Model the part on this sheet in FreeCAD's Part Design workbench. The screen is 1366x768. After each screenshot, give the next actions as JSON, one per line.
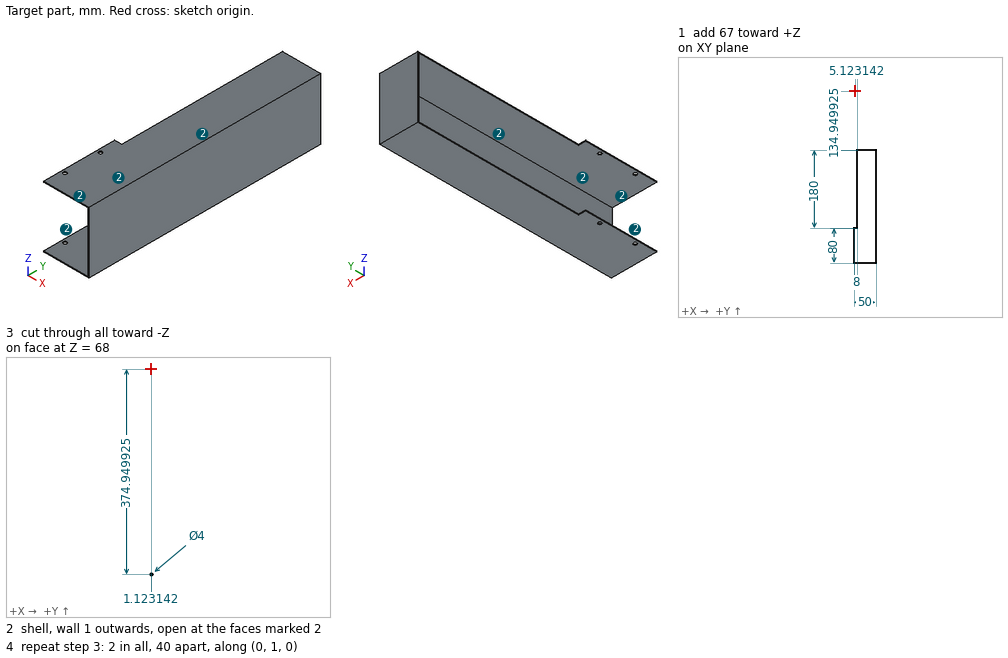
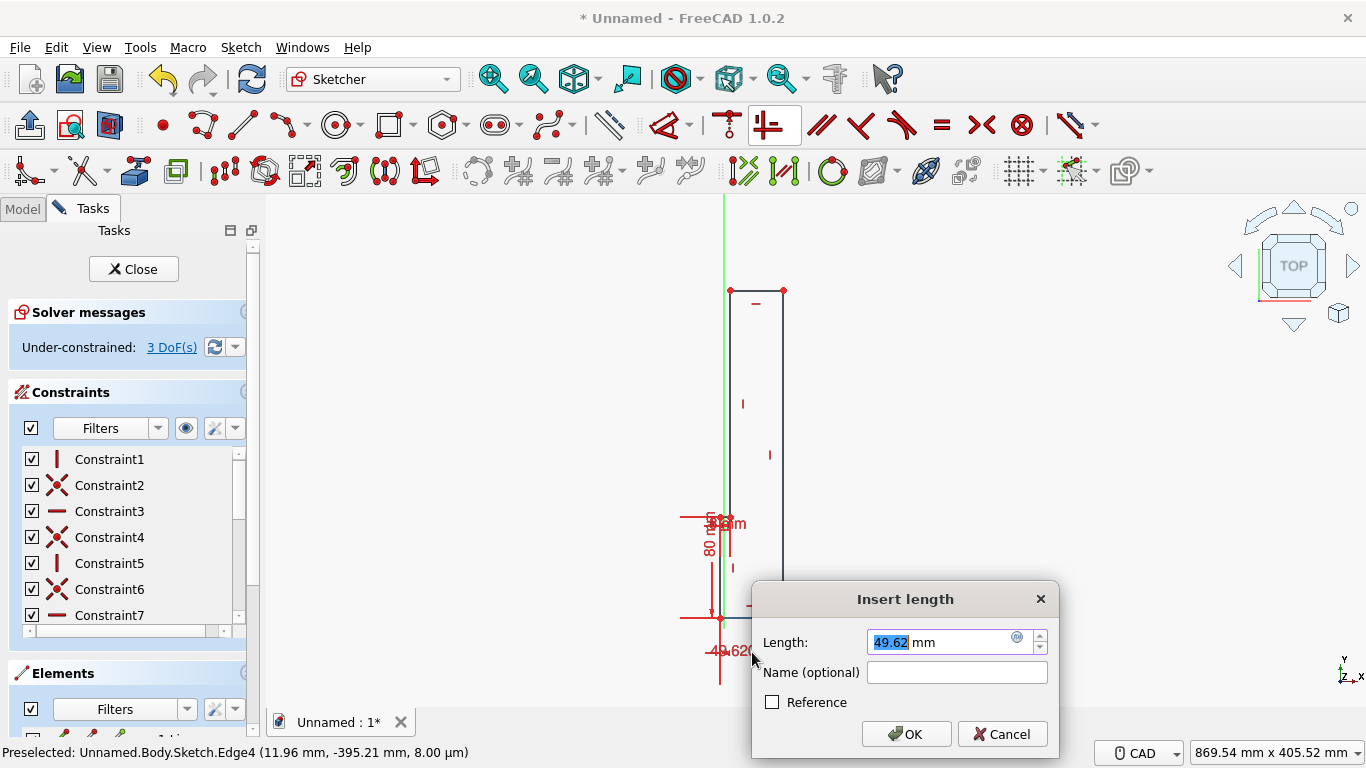
{"action": "type", "text": "50"}
{"action": "key", "text": "Return"}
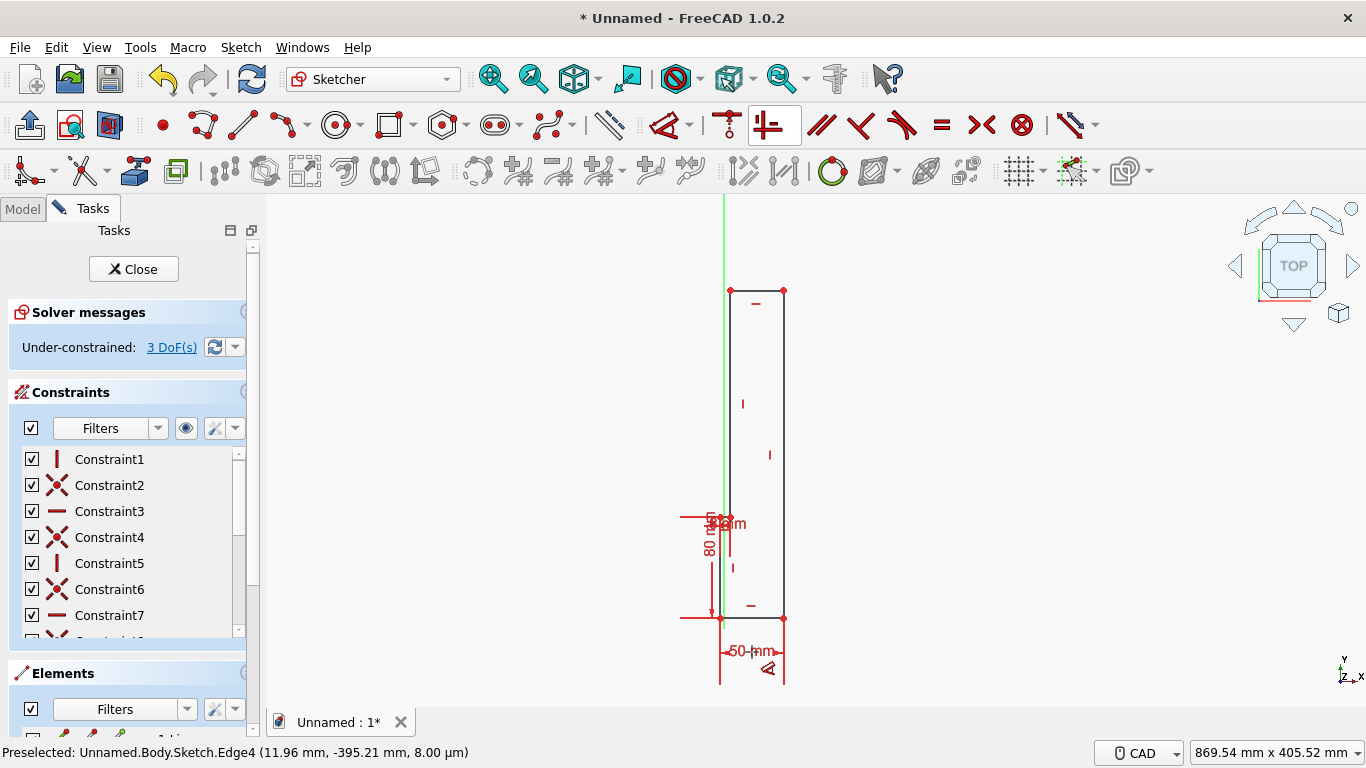
{"action": "scroll", "coordinate": [730, 359], "scroll_direction": "up", "scroll_amount": 4}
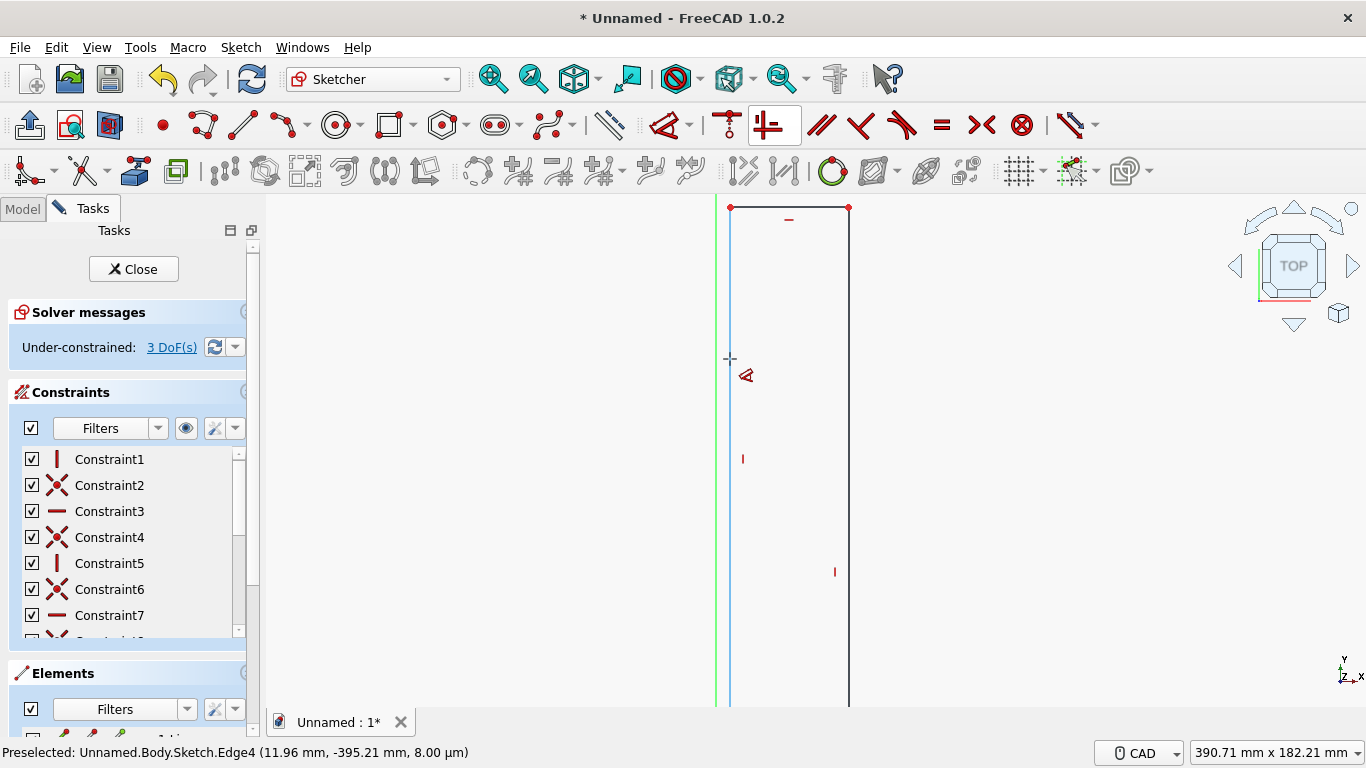
{"action": "left_click", "coordinate": [730, 358]}
{"action": "left_click", "coordinate": [696, 450]}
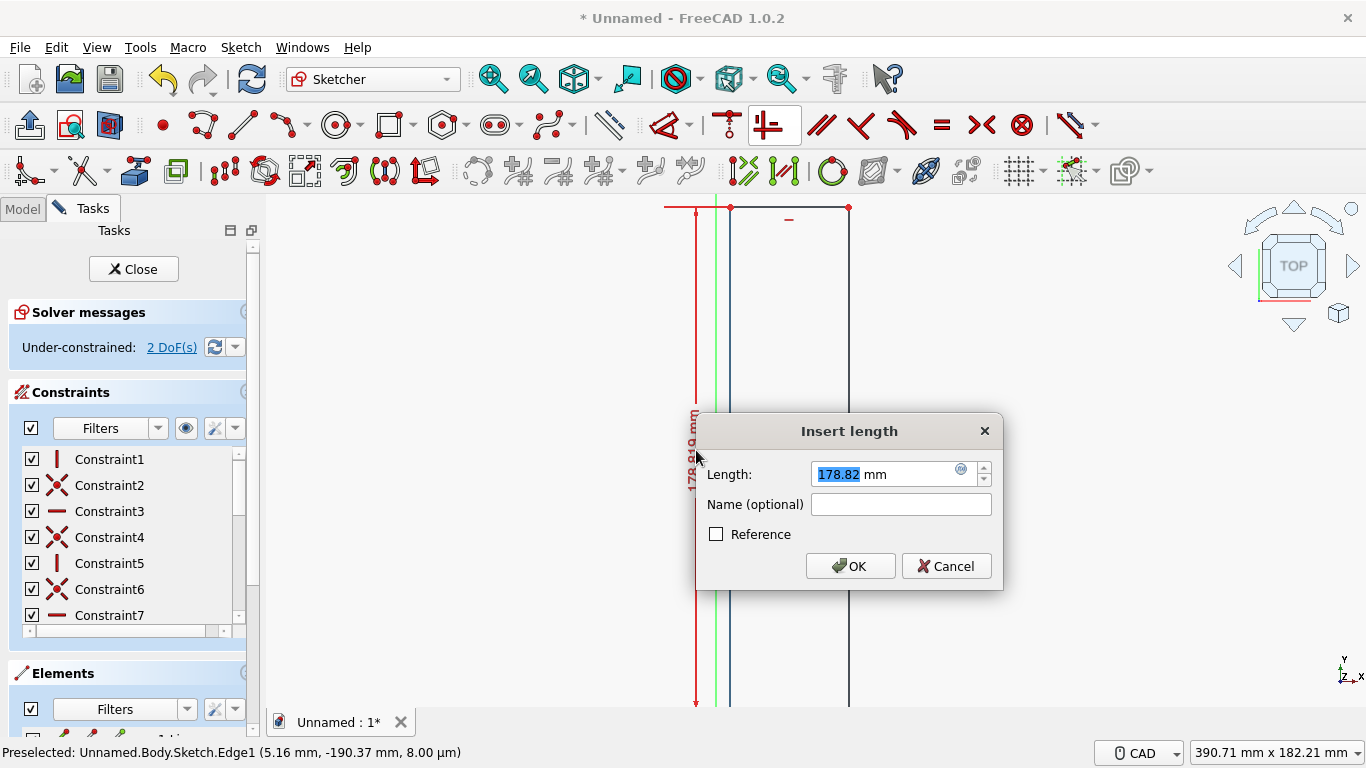
{"action": "type", "text": "180"}
{"action": "key", "text": "Return"}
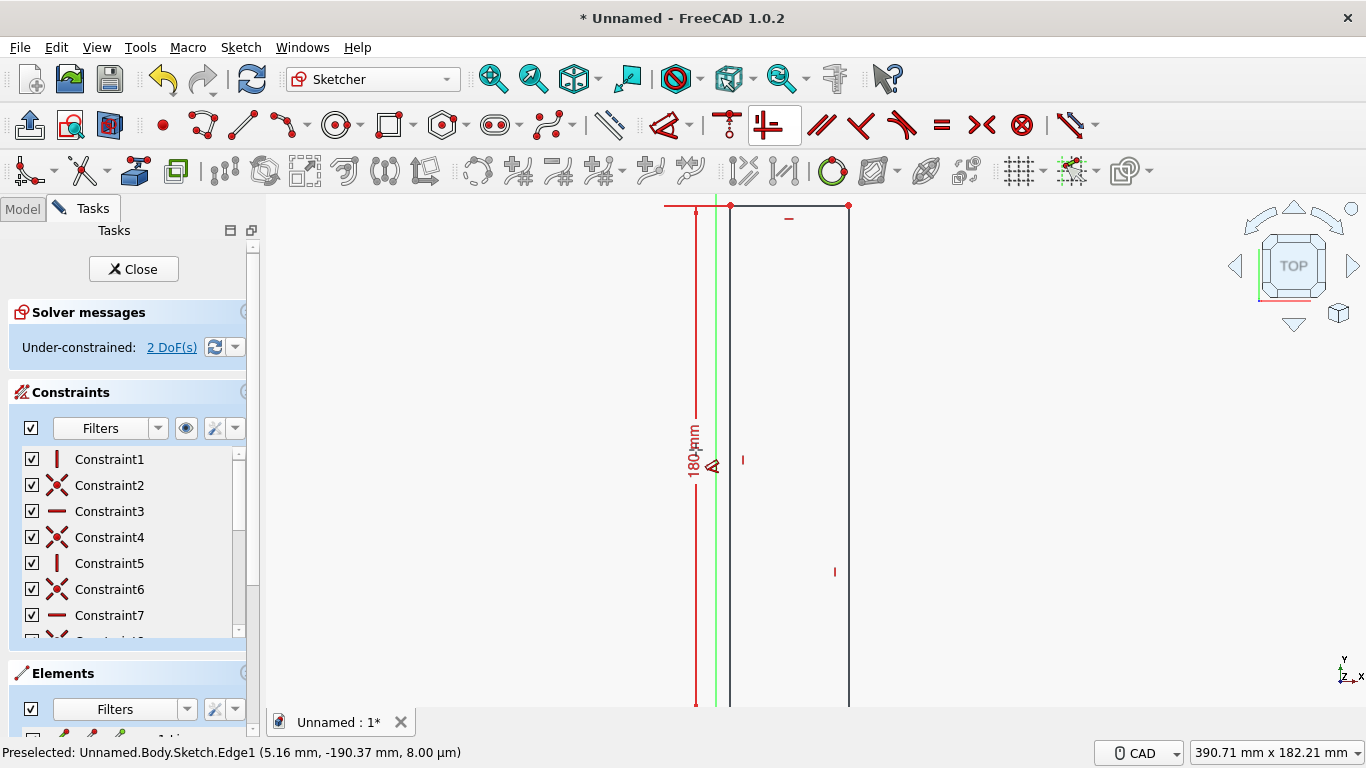
{"action": "scroll", "coordinate": [734, 481], "scroll_direction": "down", "scroll_amount": 6}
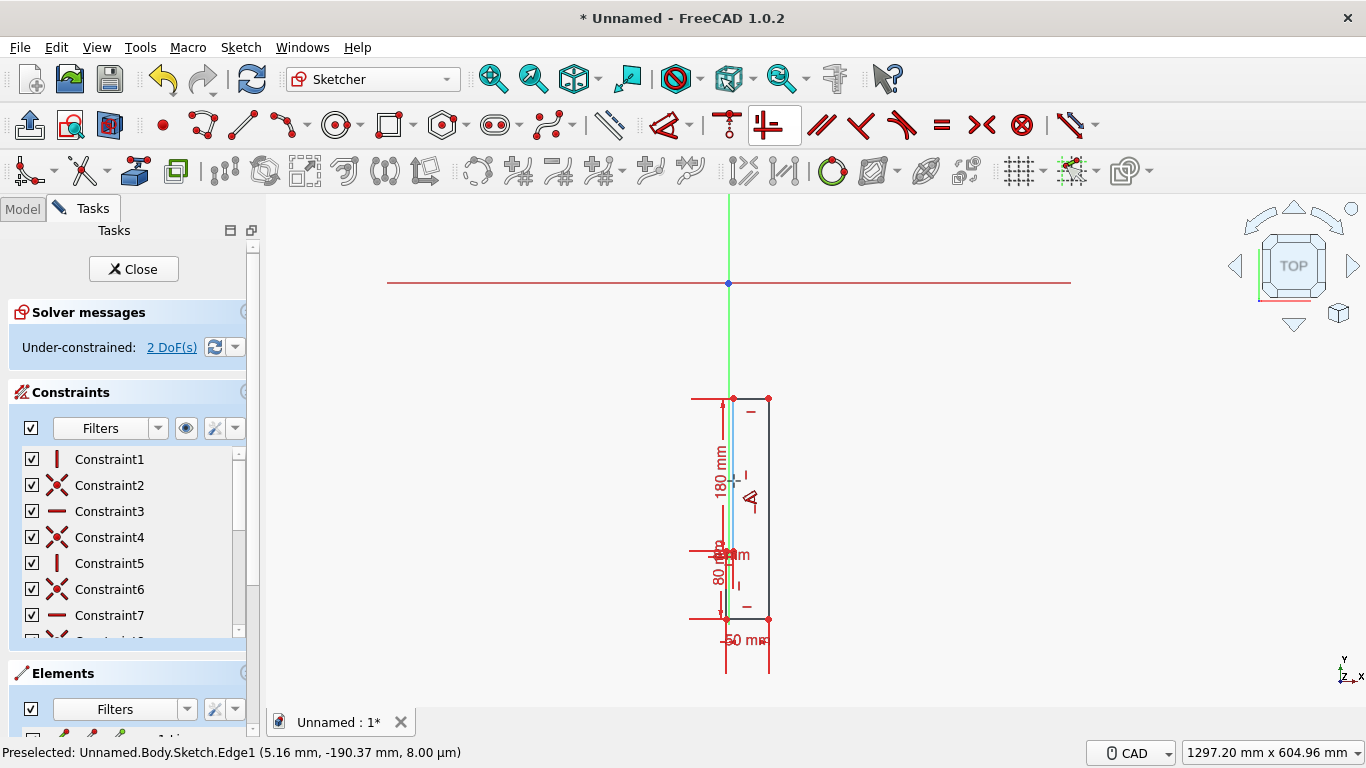
{"action": "scroll", "coordinate": [733, 399], "scroll_direction": "up", "scroll_amount": 12}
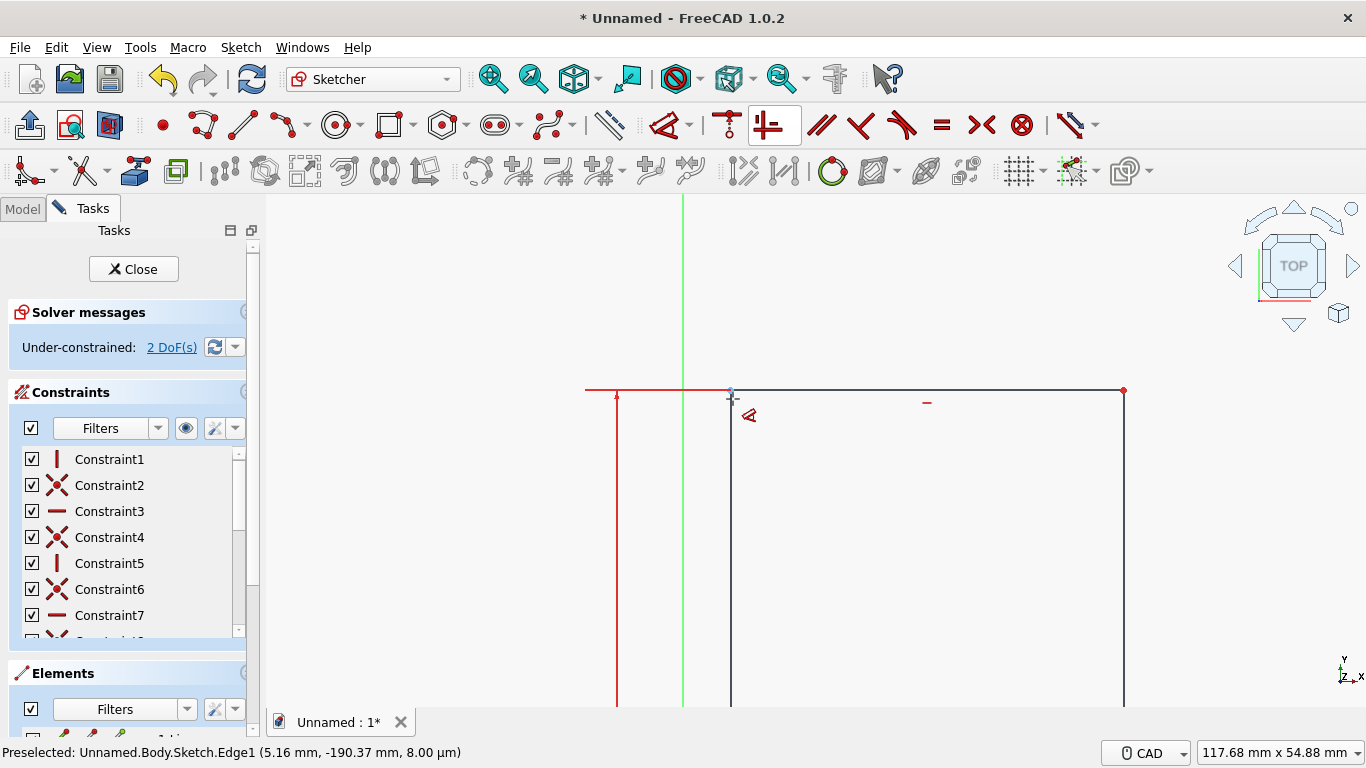
{"action": "left_click", "coordinate": [731, 390]}
{"action": "left_click", "coordinate": [707, 424]}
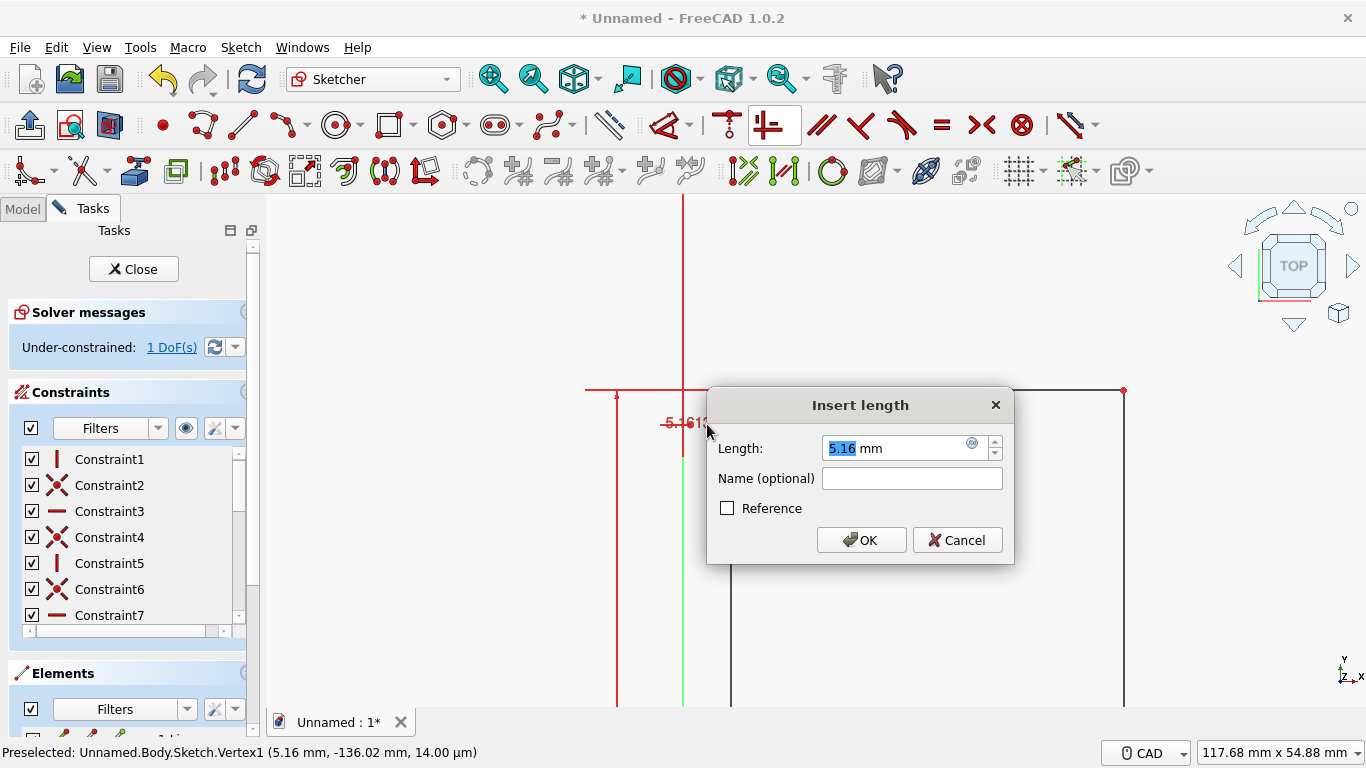
{"action": "type", "text": "5.123142"}
{"action": "key", "text": "Return"}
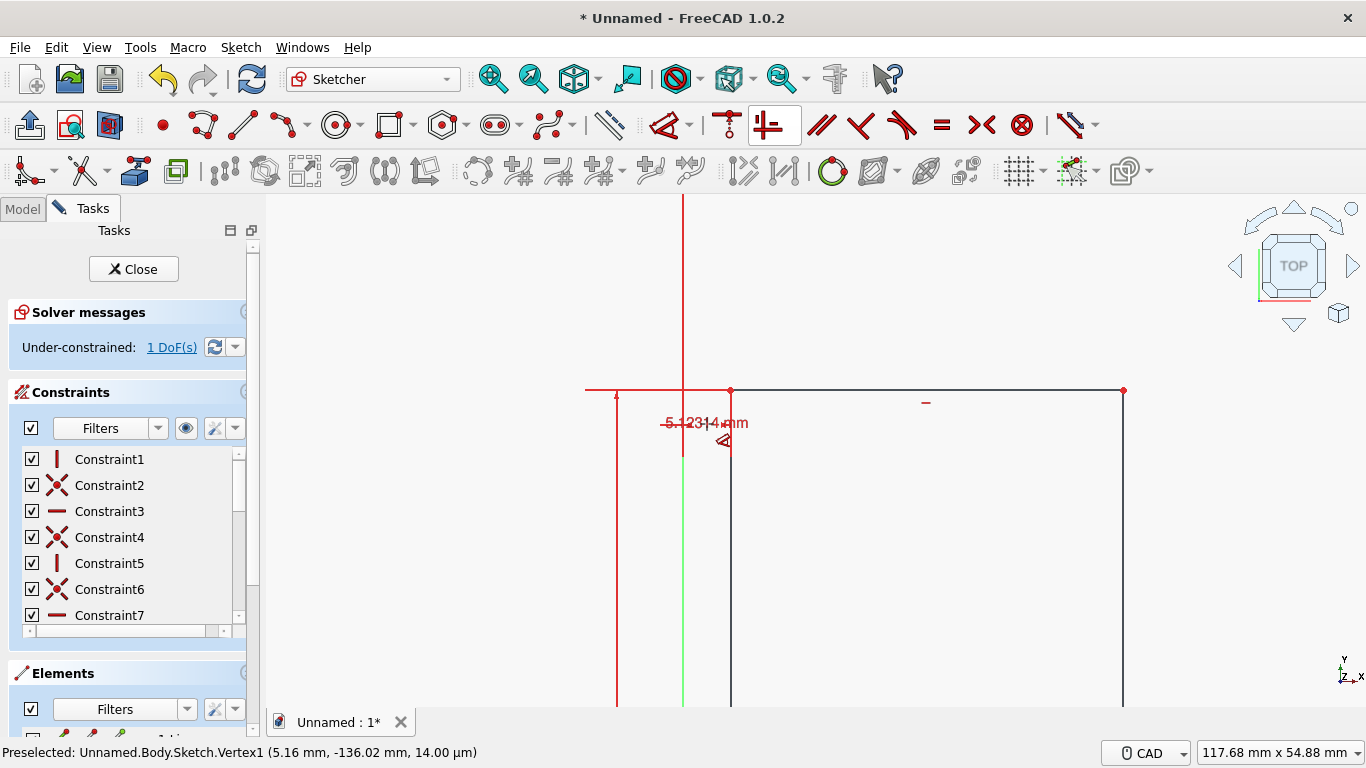
{"action": "scroll", "coordinate": [733, 399], "scroll_direction": "down", "scroll_amount": 12}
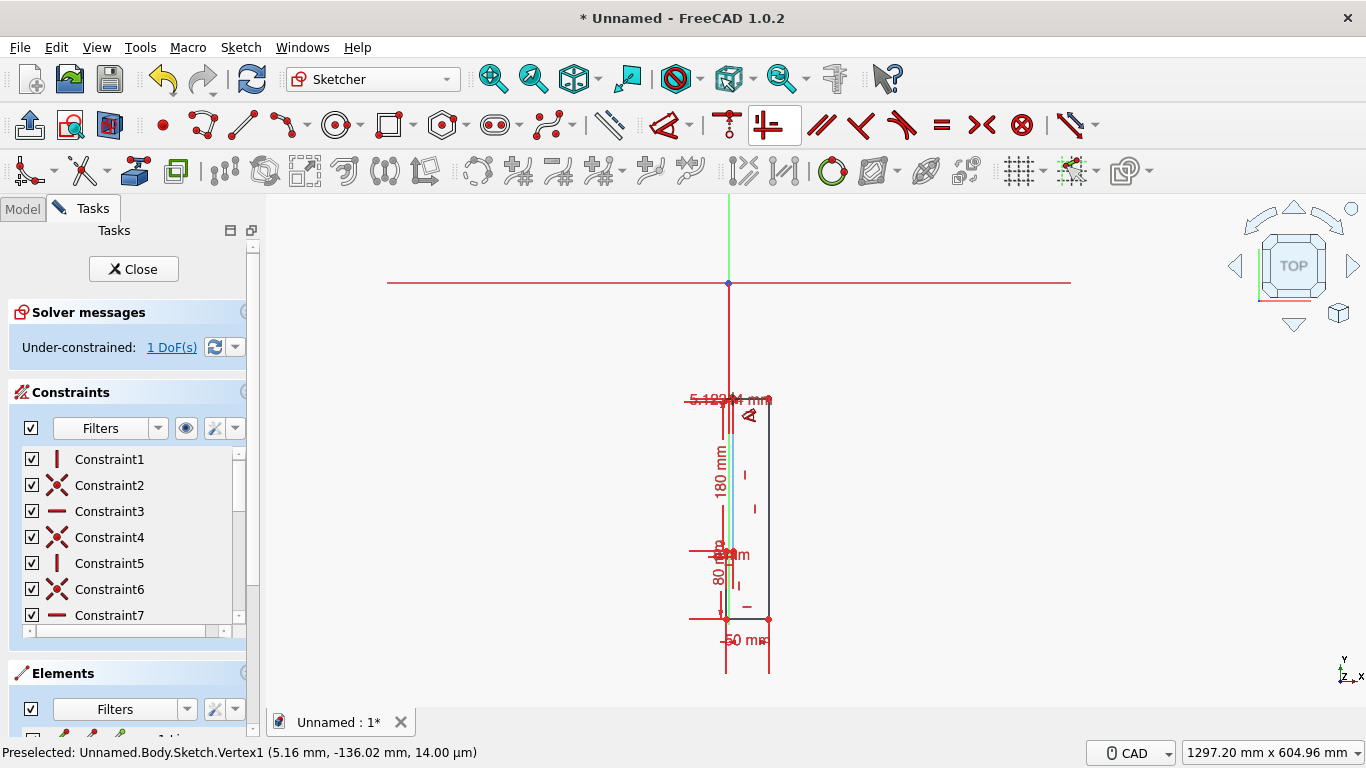
{"action": "left_click", "coordinate": [733, 399]}
{"action": "left_click", "coordinate": [695, 341]}